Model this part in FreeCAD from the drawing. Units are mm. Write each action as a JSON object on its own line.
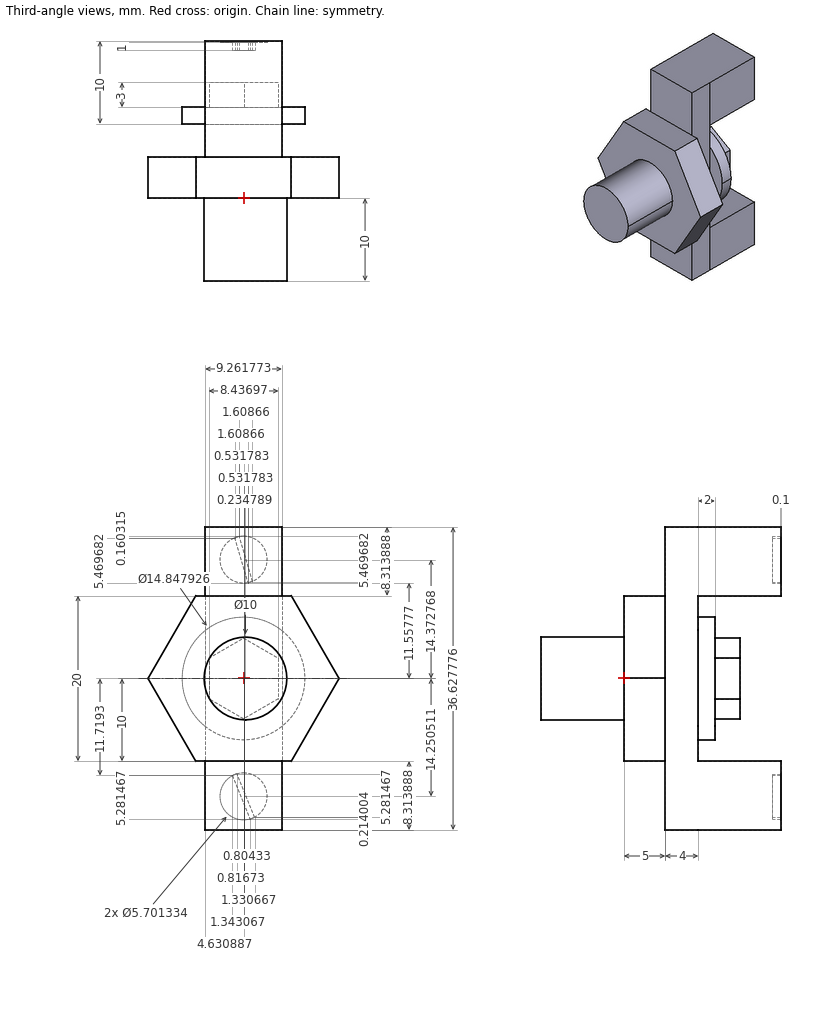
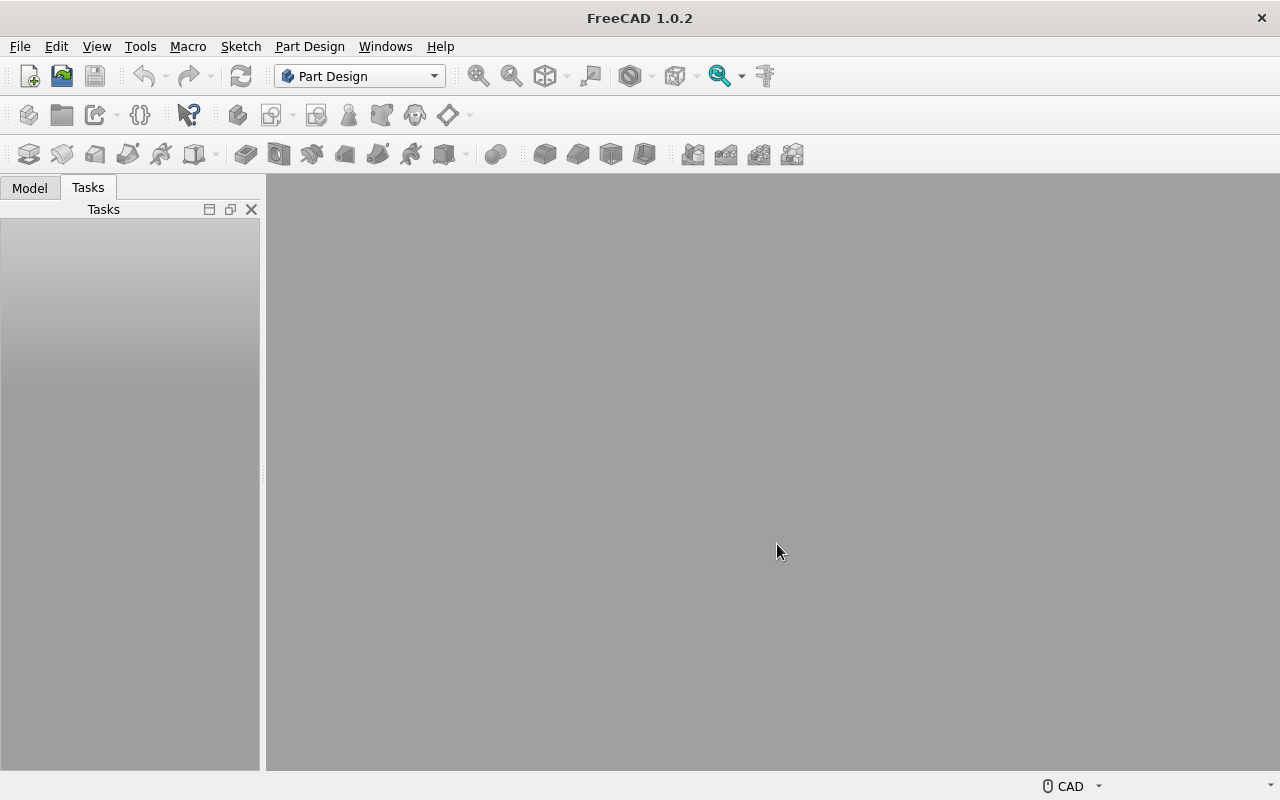
{"action": "left_click", "coordinate": [29, 76]}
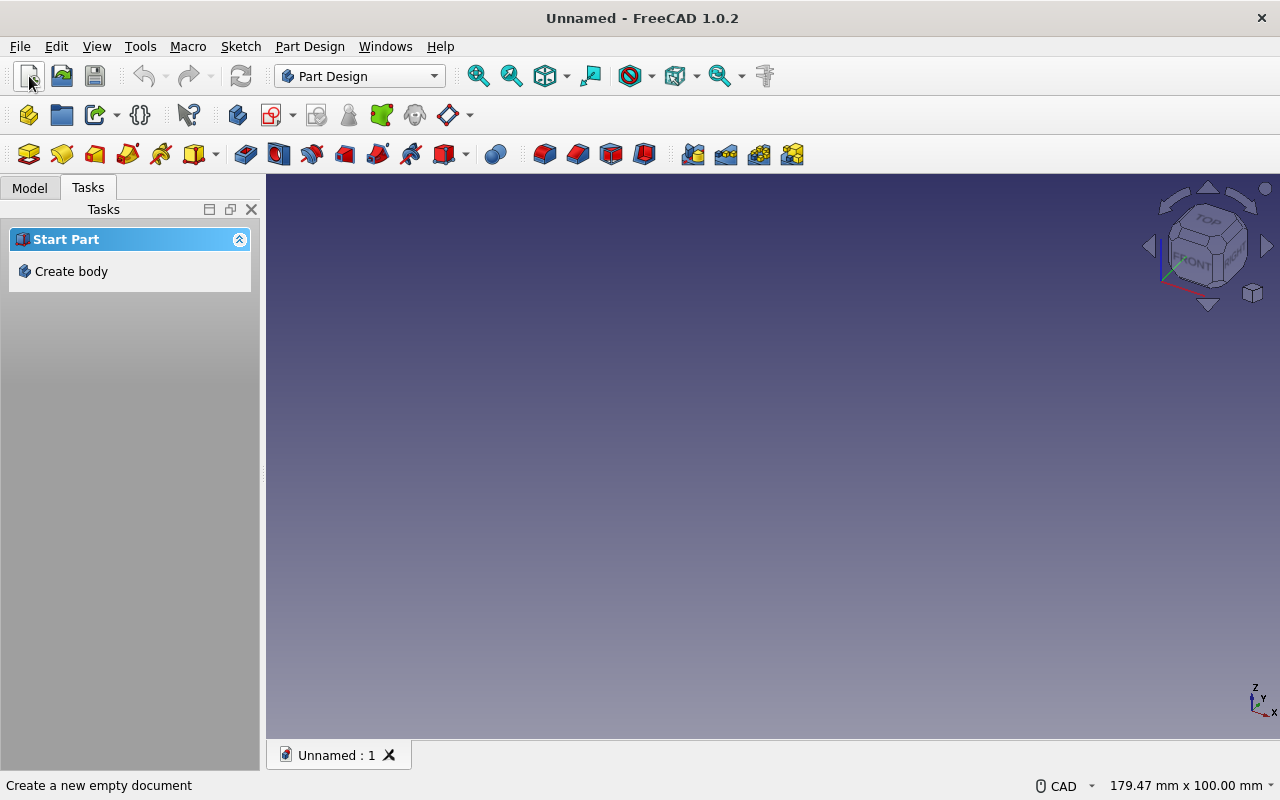
{"action": "left_click", "coordinate": [270, 116]}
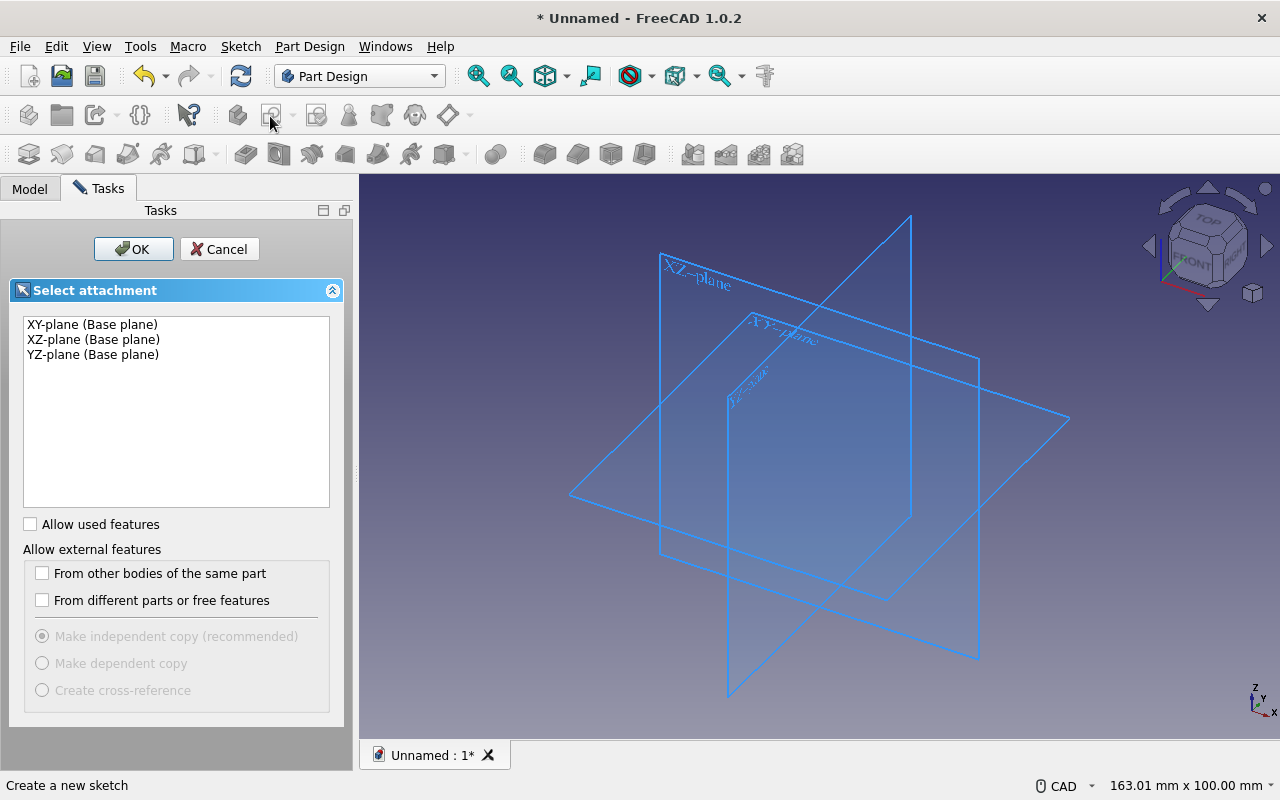
{"action": "left_click", "coordinate": [84, 340]}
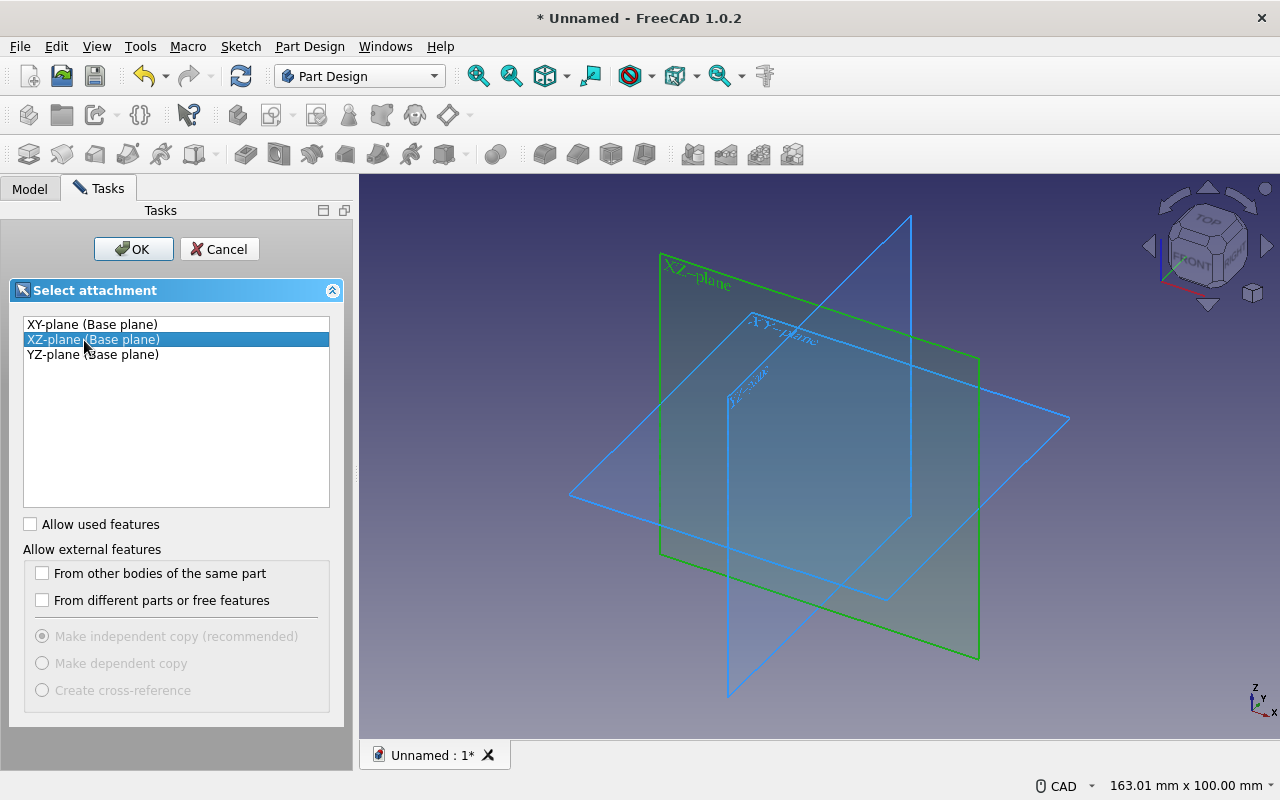
{"action": "left_click", "coordinate": [134, 249]}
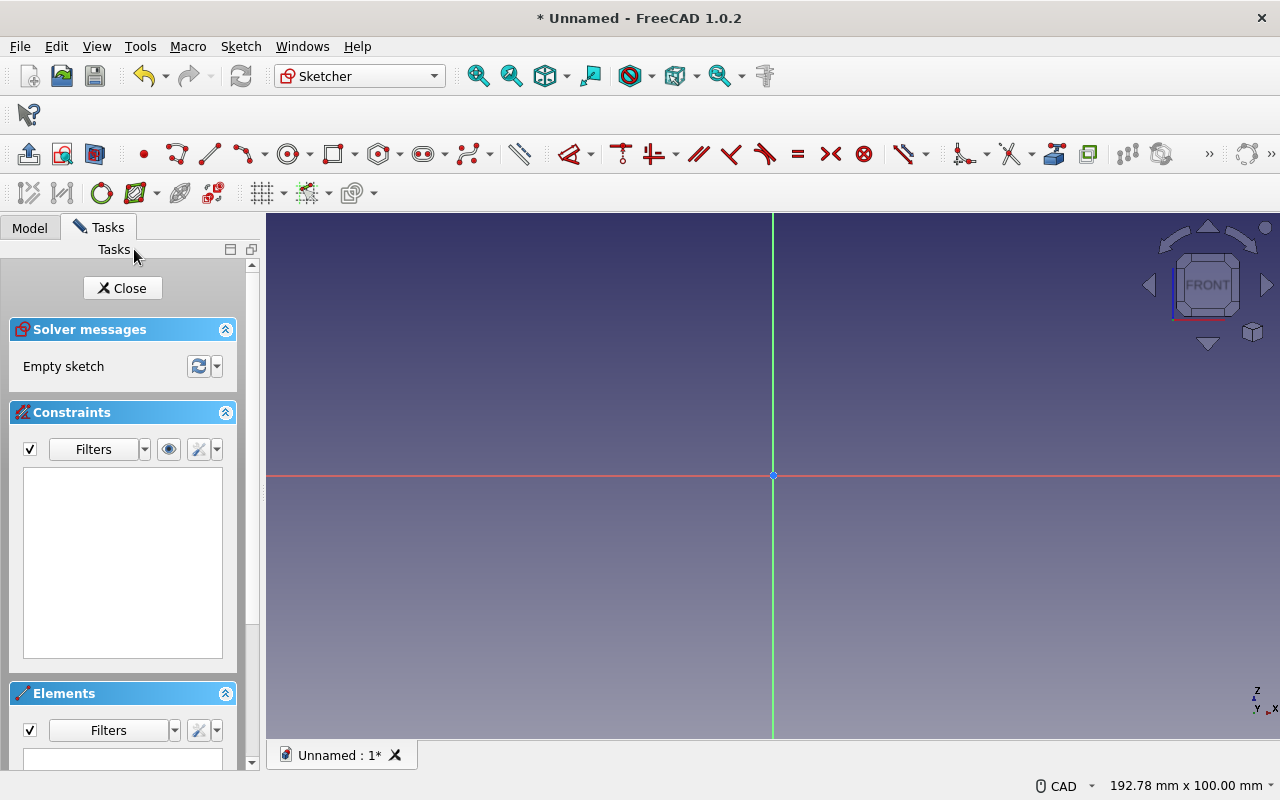
{"action": "scroll", "coordinate": [803, 476], "scroll_direction": "up", "scroll_amount": 6}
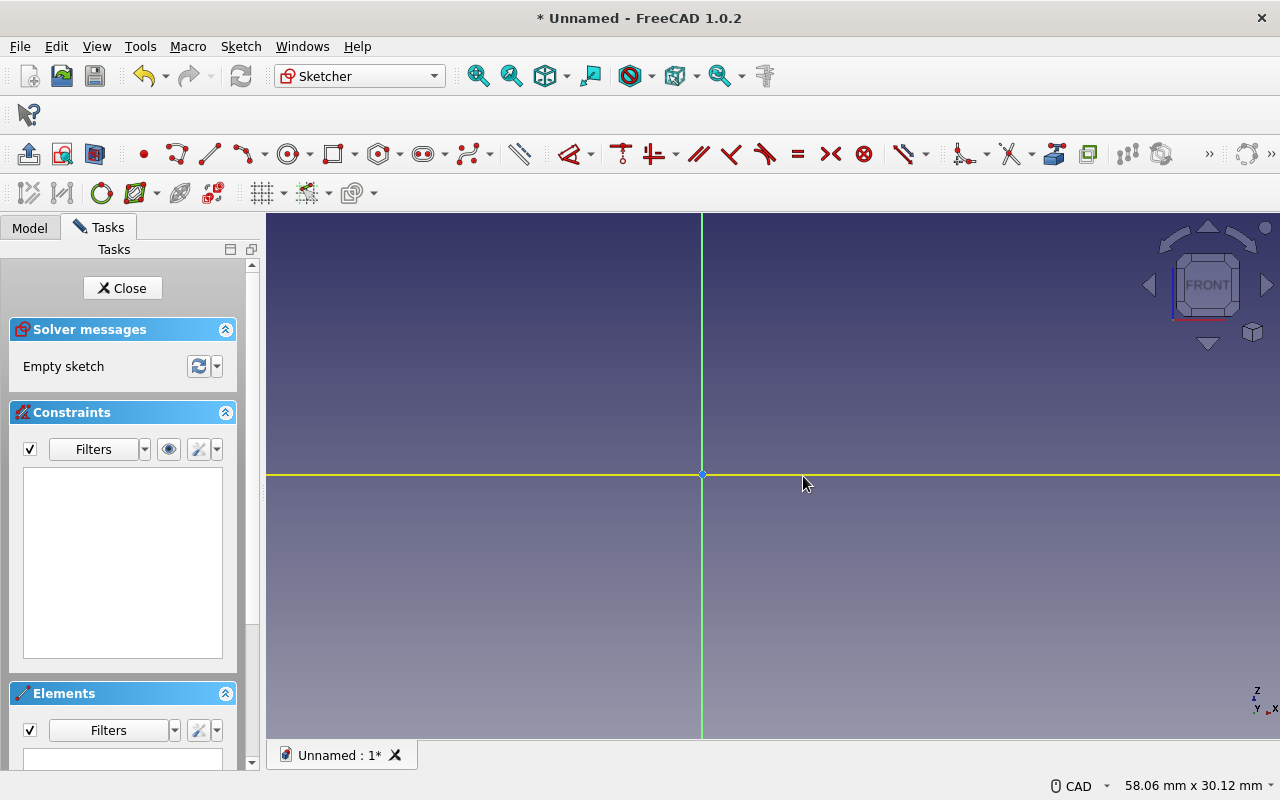
{"action": "left_click", "coordinate": [378, 154]}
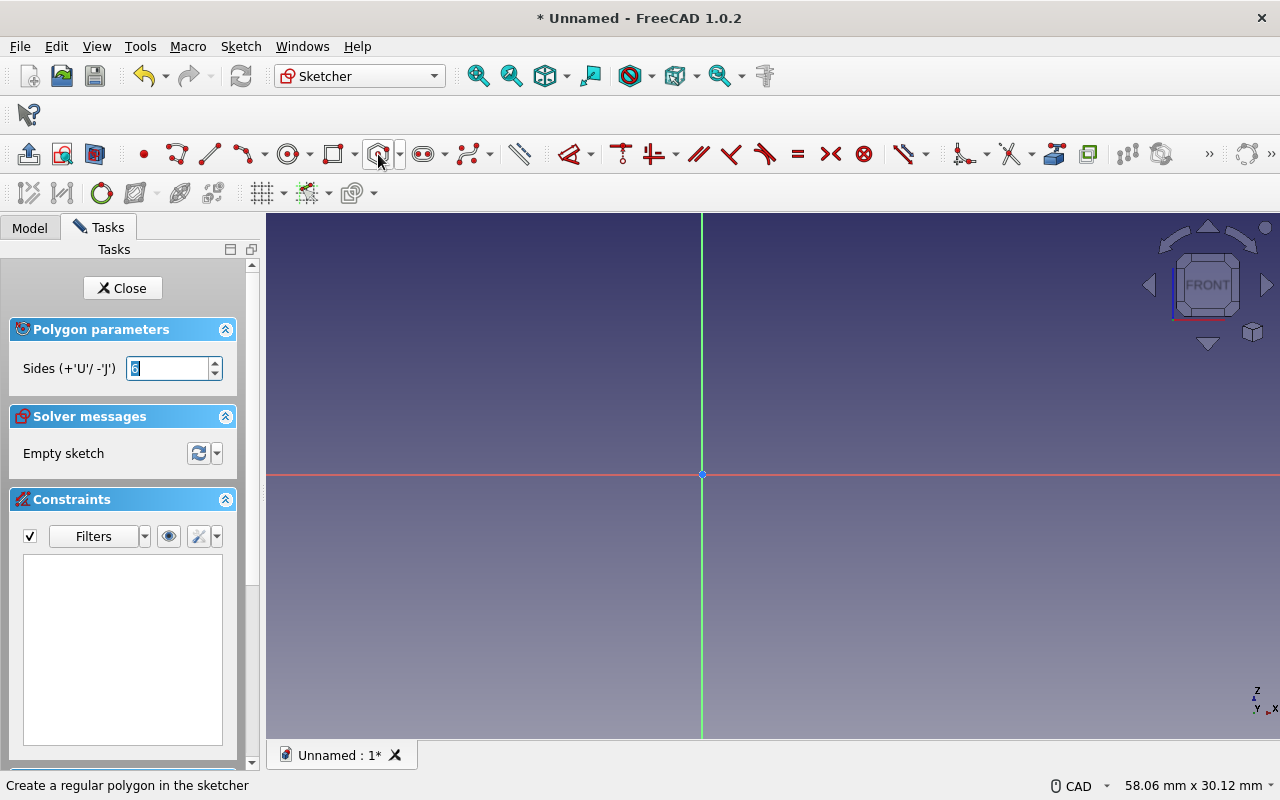
{"action": "left_click", "coordinate": [702, 475]}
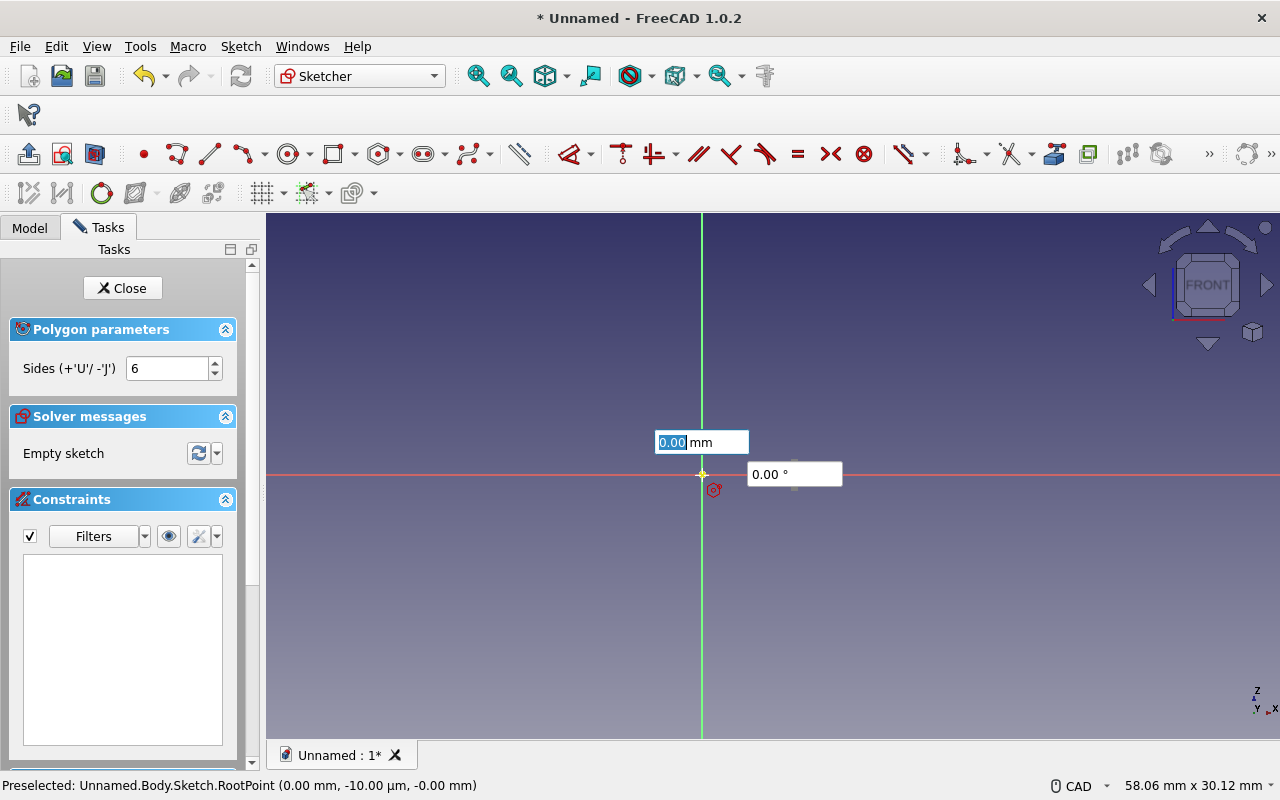
{"action": "left_click", "coordinate": [501, 475]}
{"action": "key", "text": "Escape"}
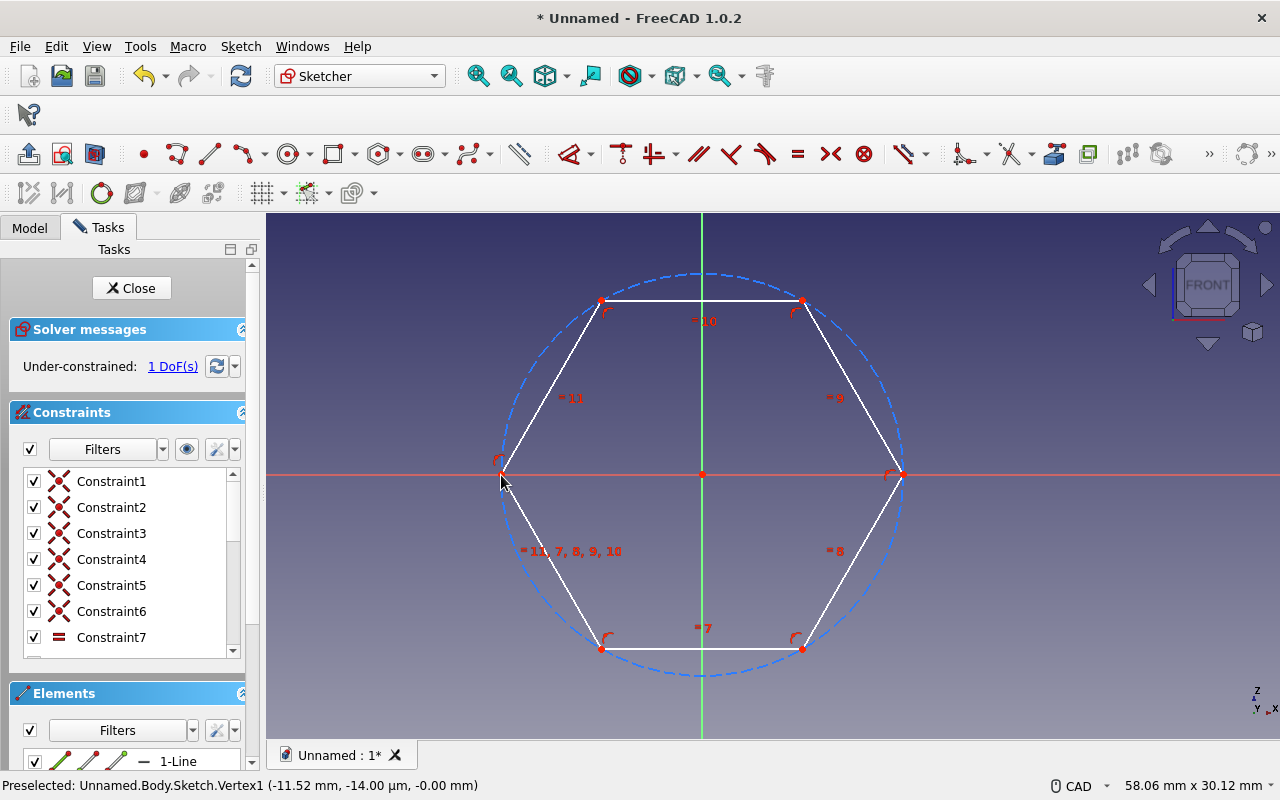
{"action": "left_click", "coordinate": [568, 154]}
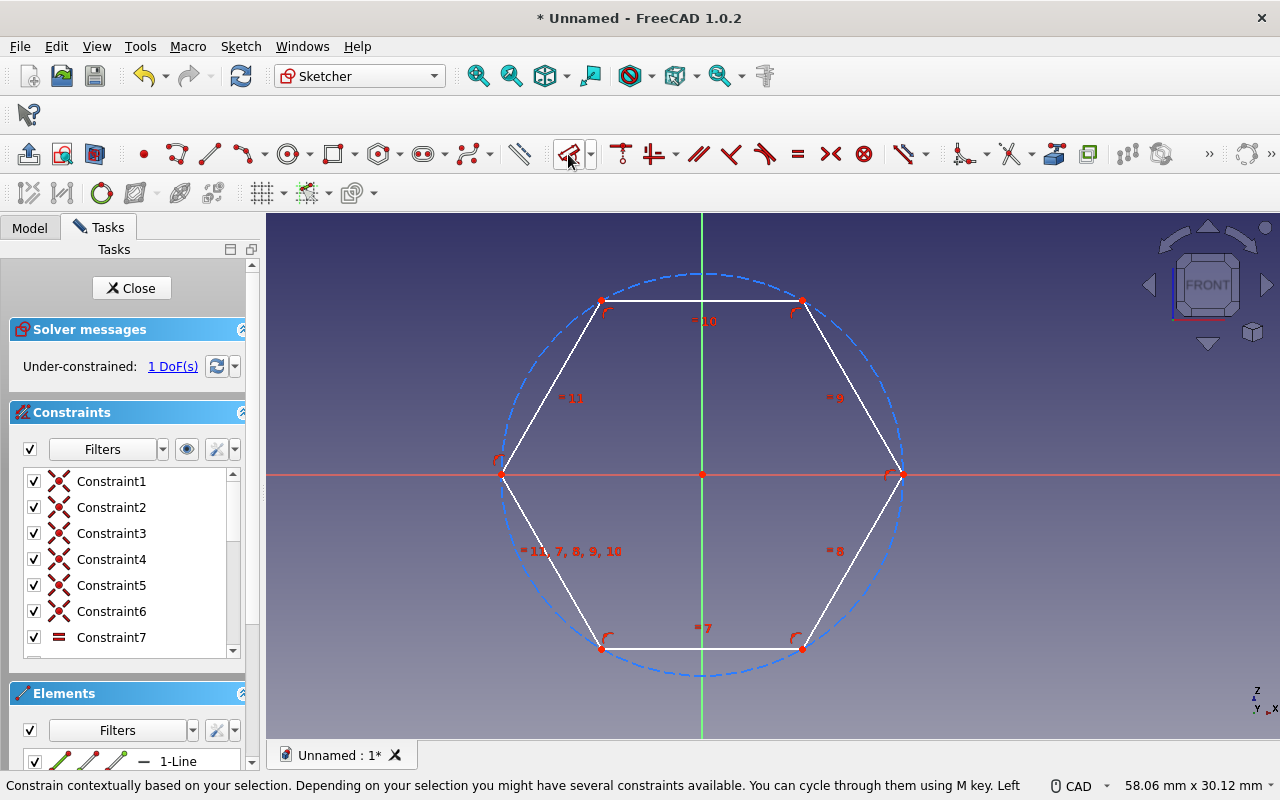
{"action": "left_click", "coordinate": [602, 649]}